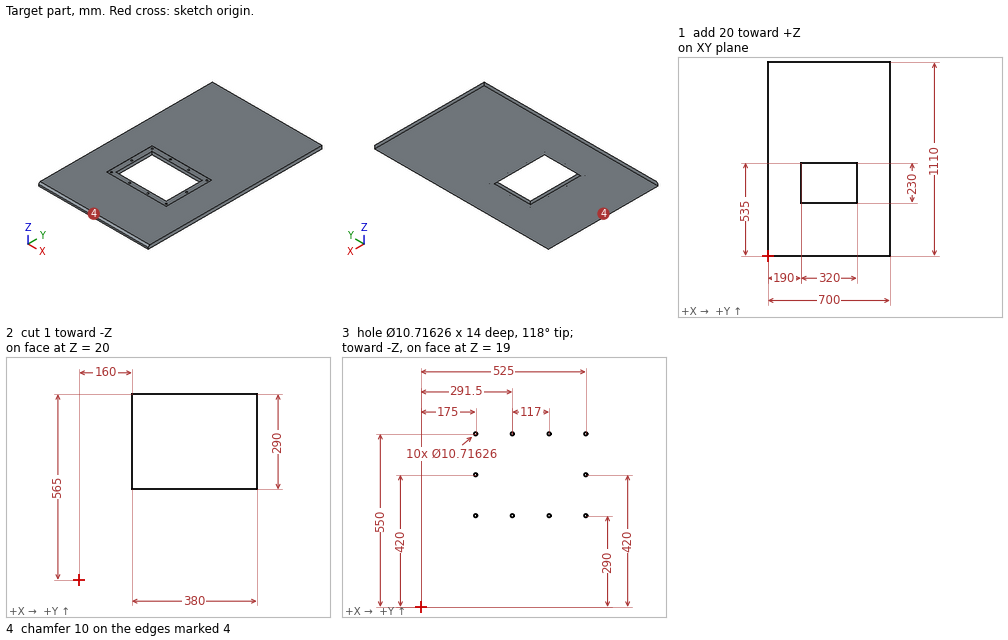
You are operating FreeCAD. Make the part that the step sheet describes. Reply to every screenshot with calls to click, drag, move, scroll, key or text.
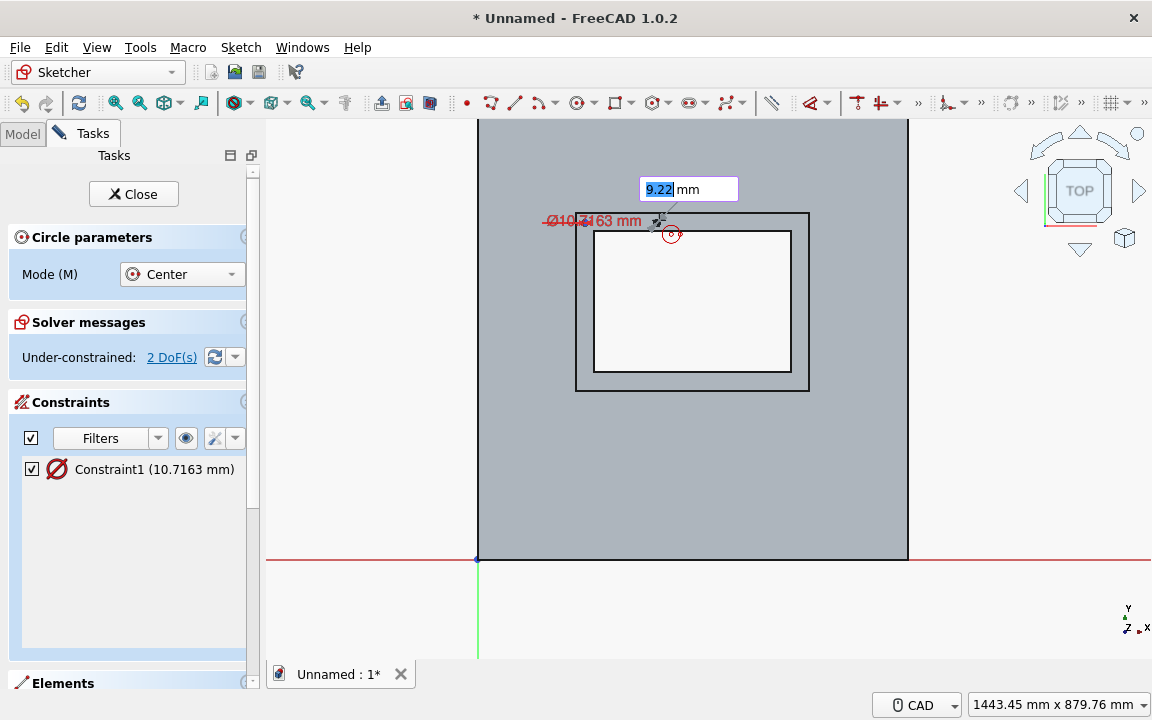
text(10.71626)
key(Return)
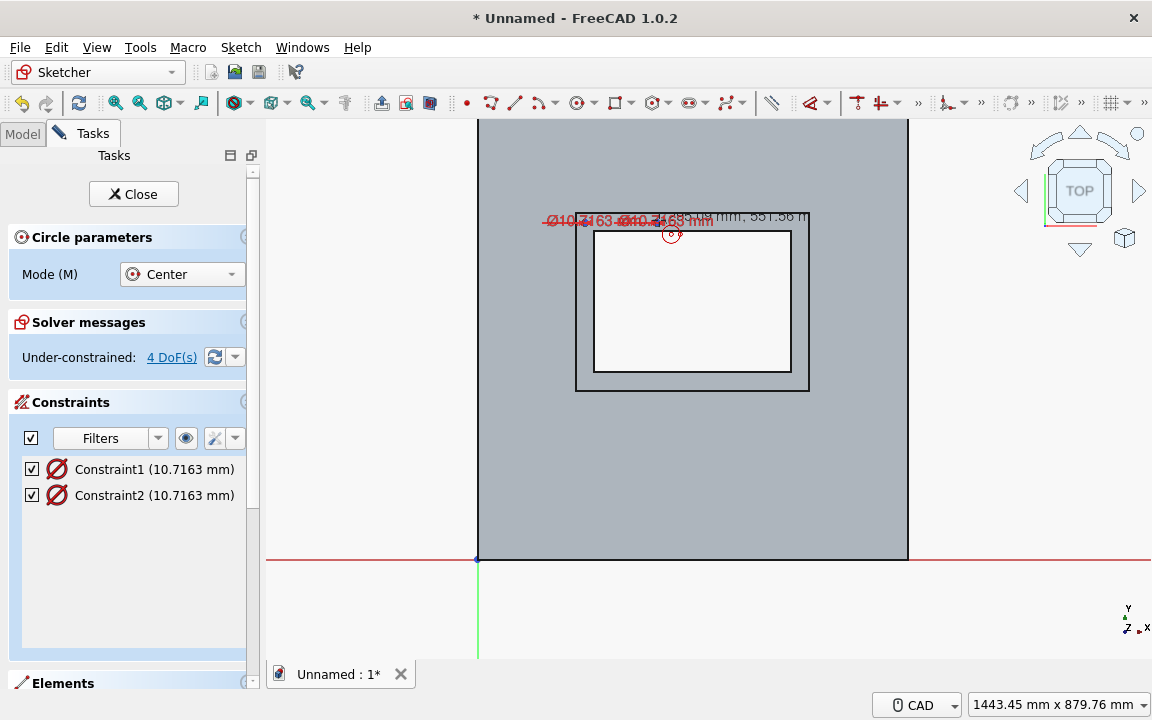
scroll(729, 222, up, 10)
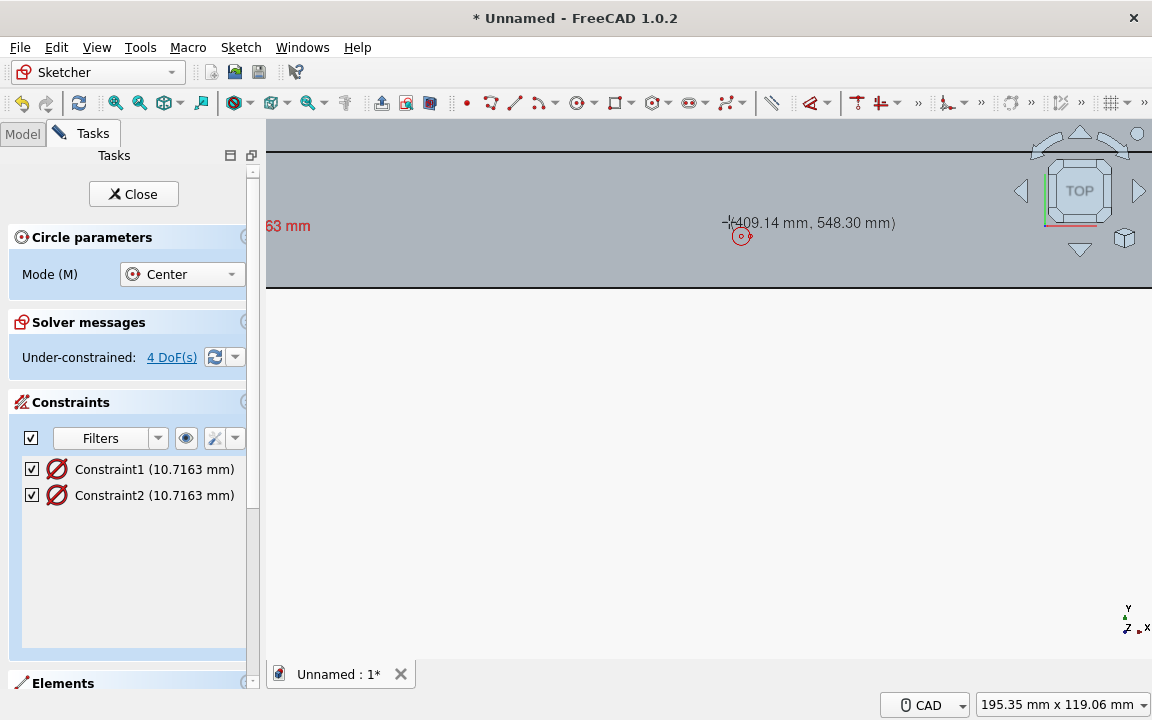
scroll(729, 222, down, 10)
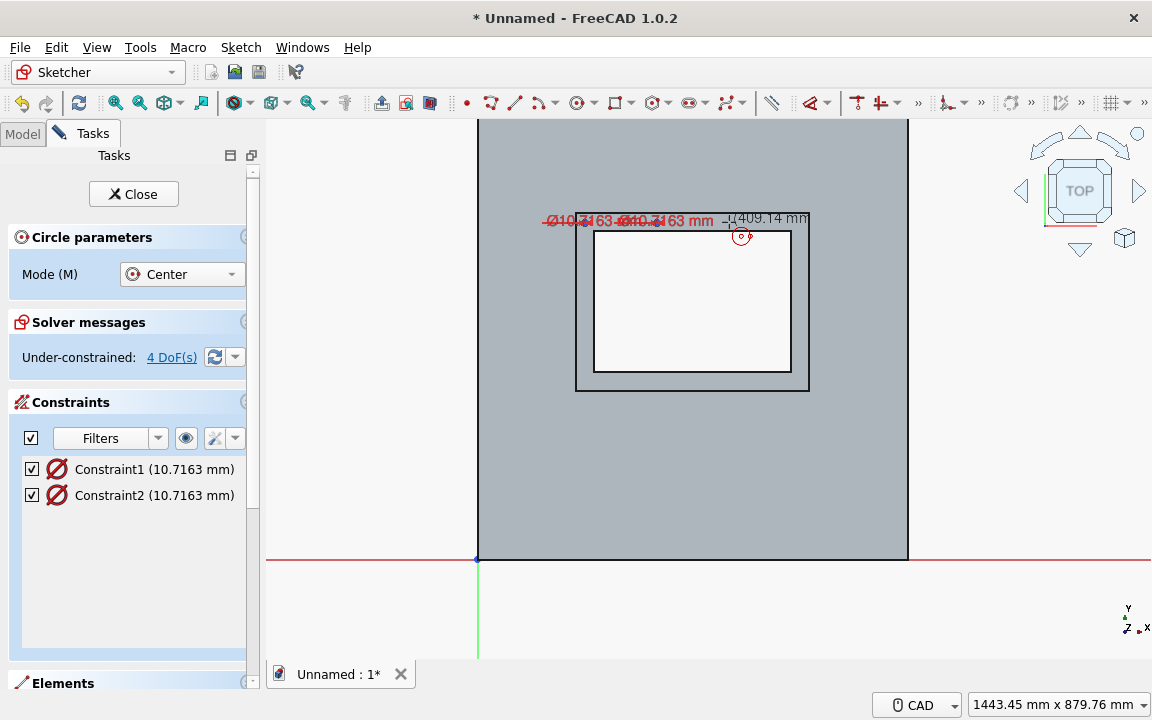
click(729, 222)
move(731, 220)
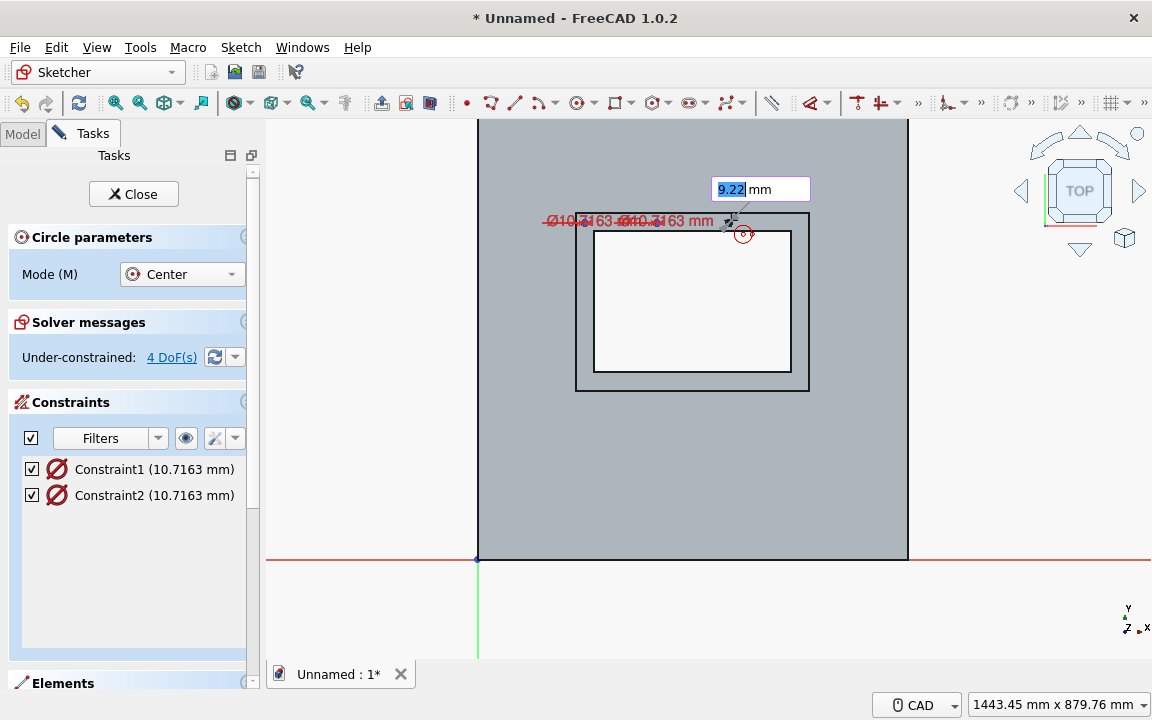
text(10.71626)
key(Return)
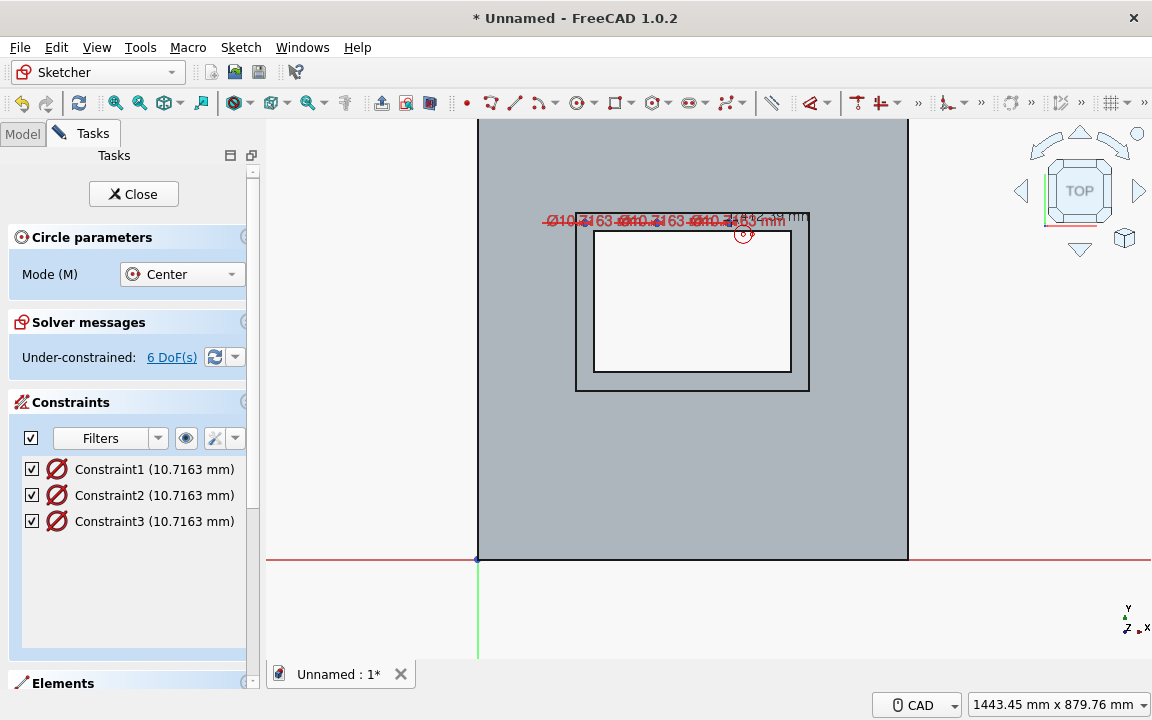
scroll(800, 222, up, 10)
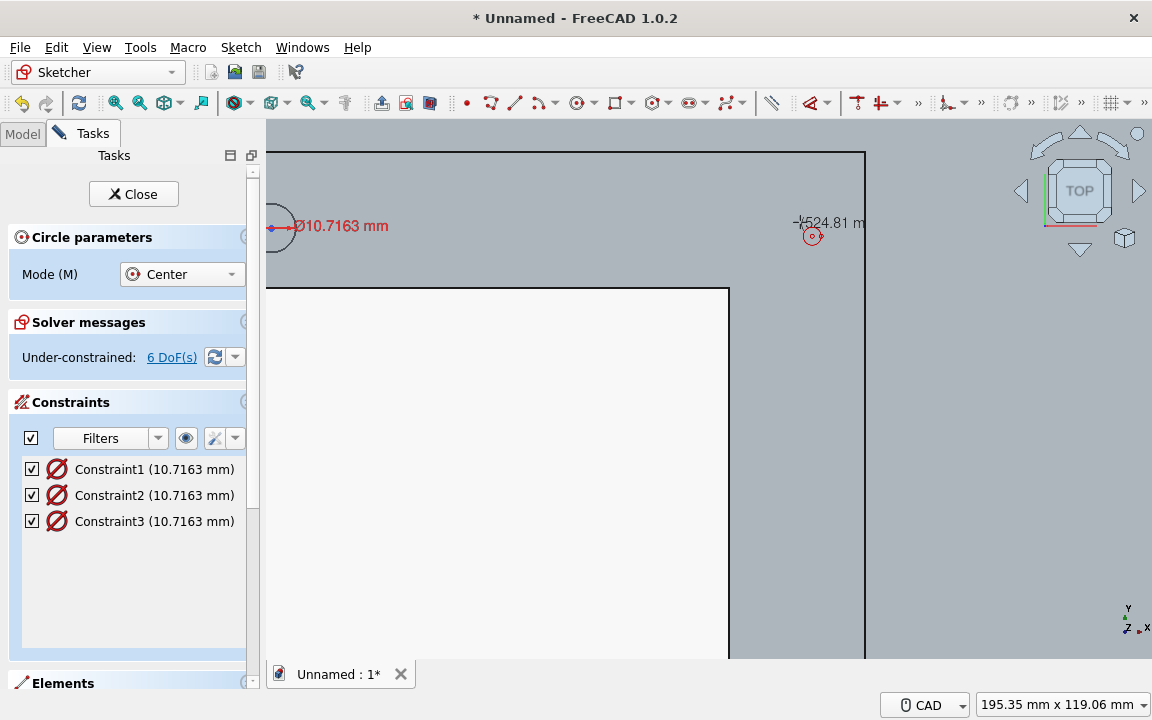
scroll(800, 222, down, 10)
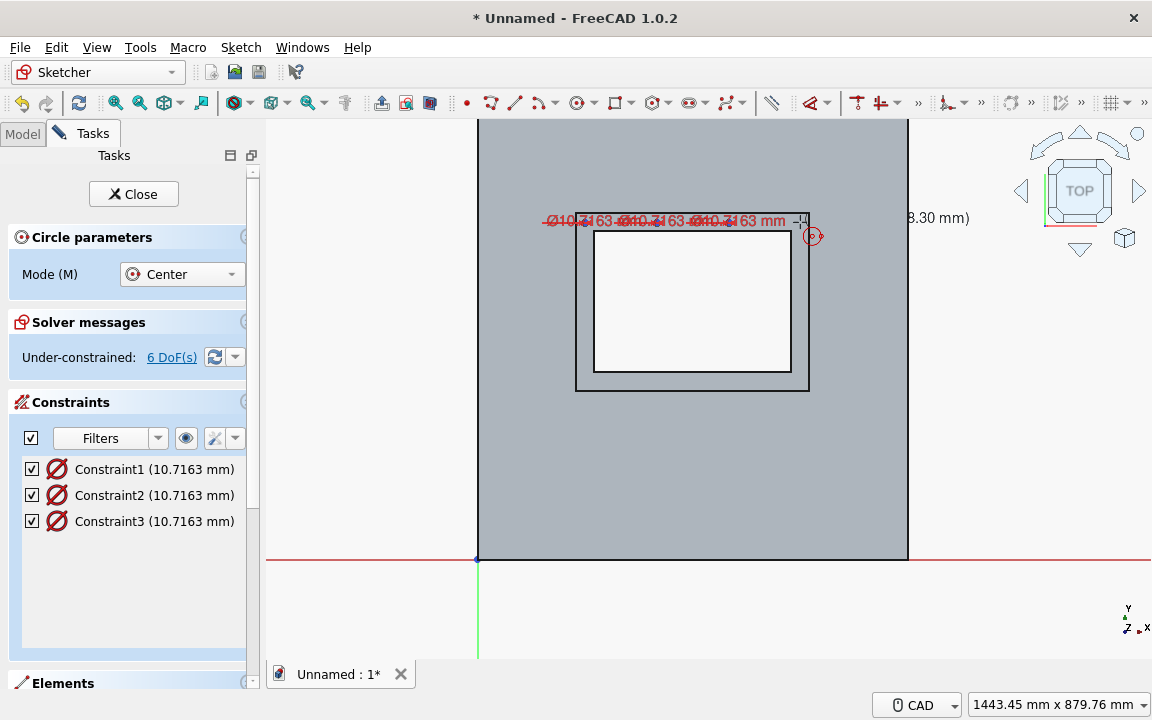
click(800, 222)
move(802, 220)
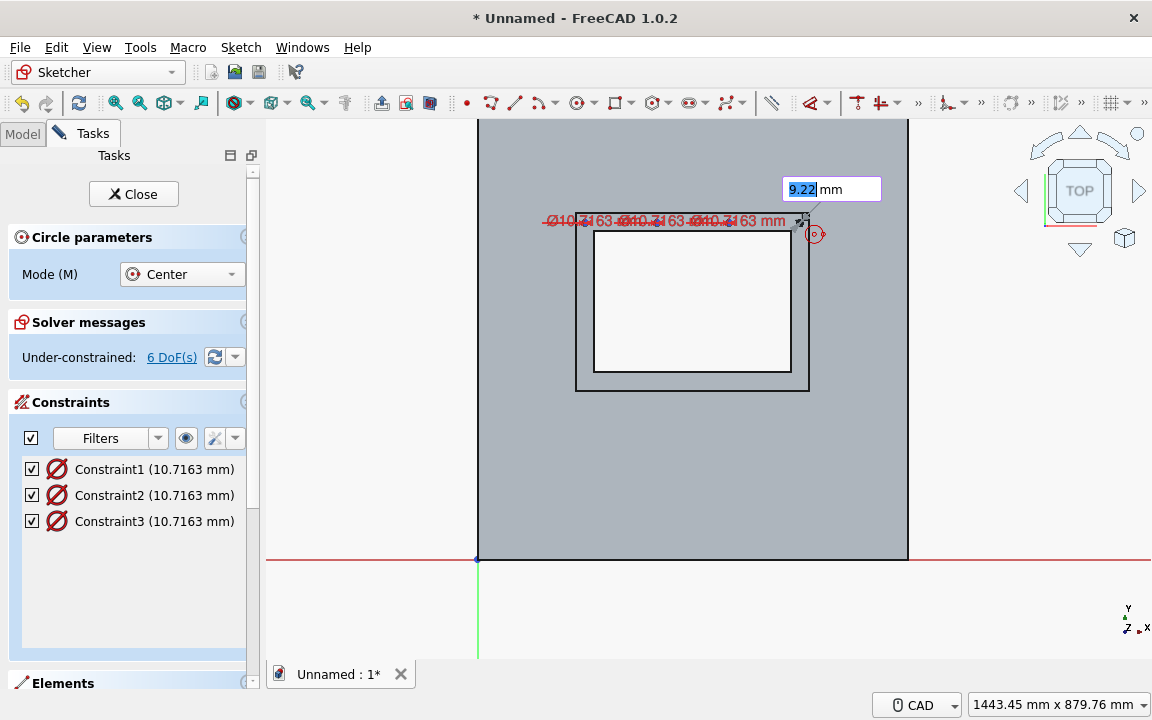
text(10.71626)
key(Return)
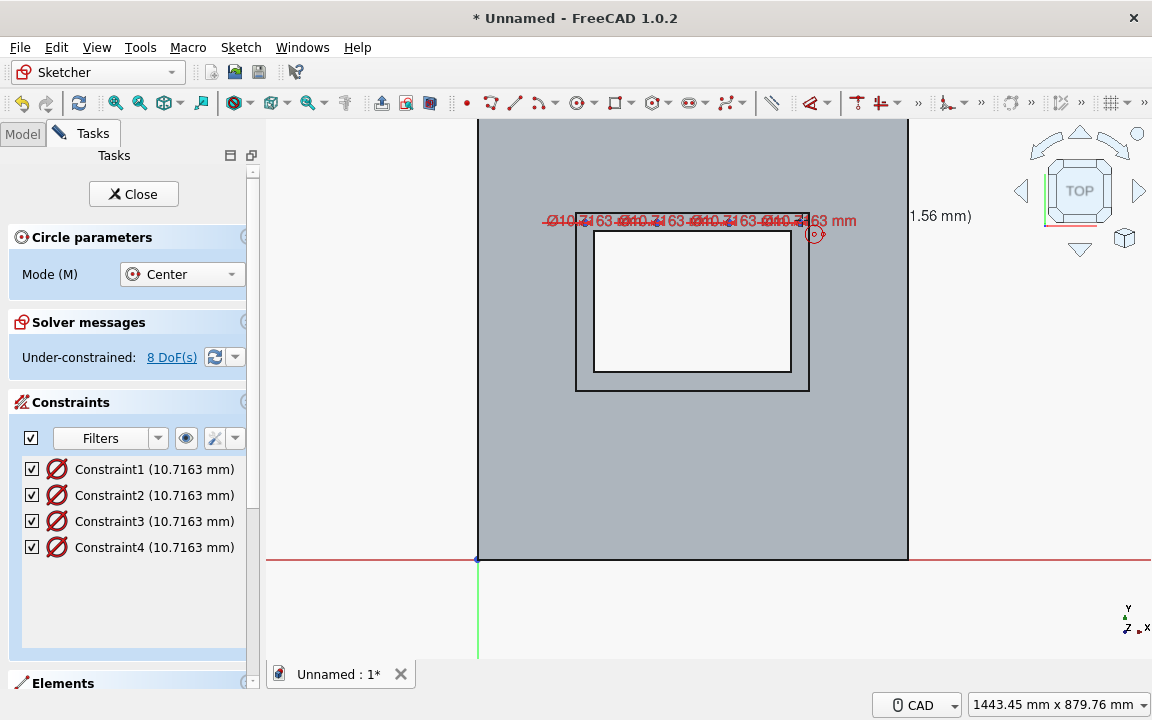
scroll(800, 302, up, 10)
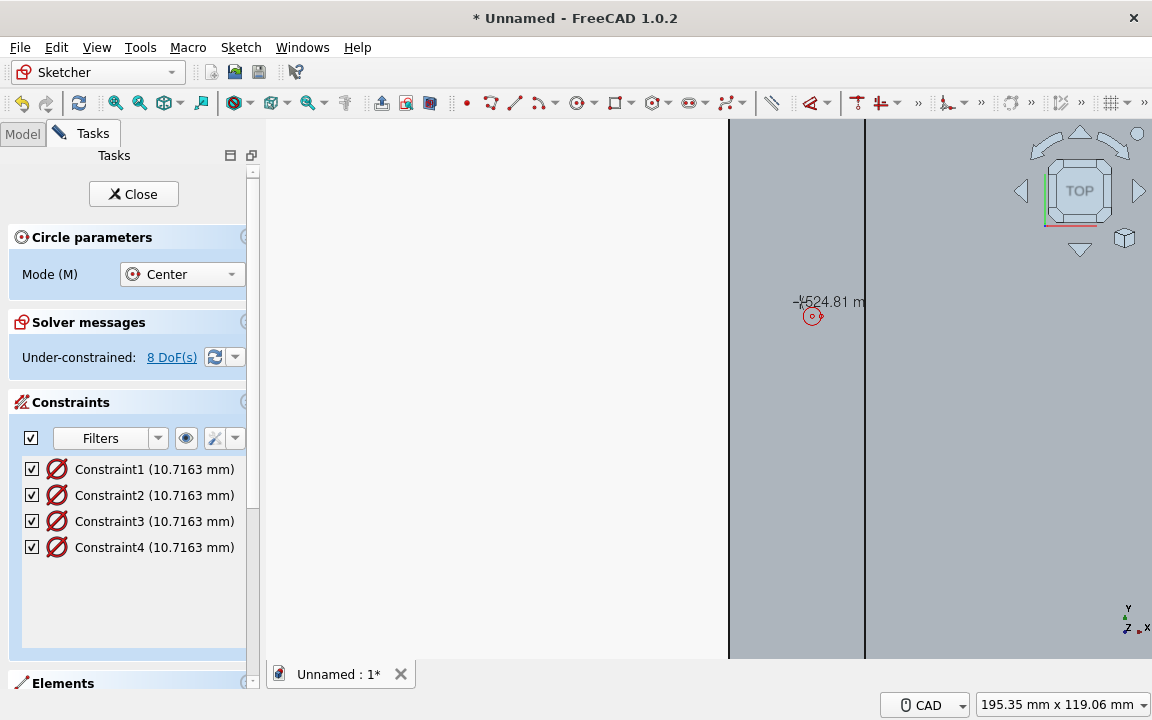
scroll(800, 302, down, 10)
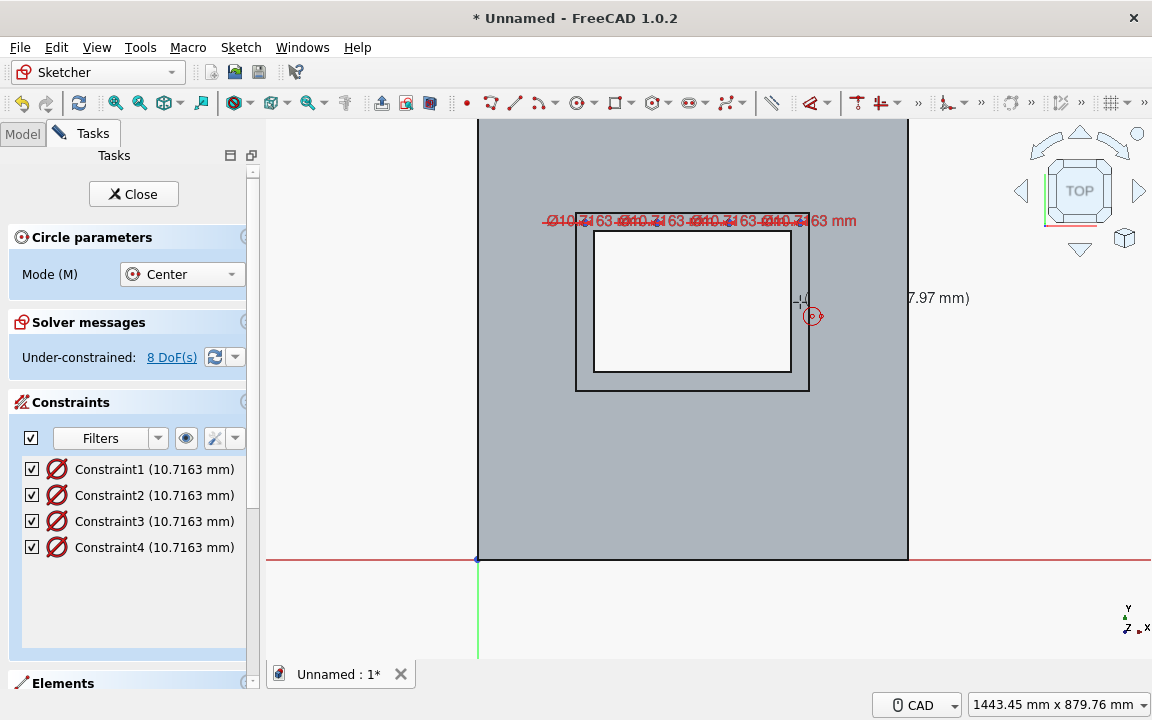
click(800, 302)
move(802, 299)